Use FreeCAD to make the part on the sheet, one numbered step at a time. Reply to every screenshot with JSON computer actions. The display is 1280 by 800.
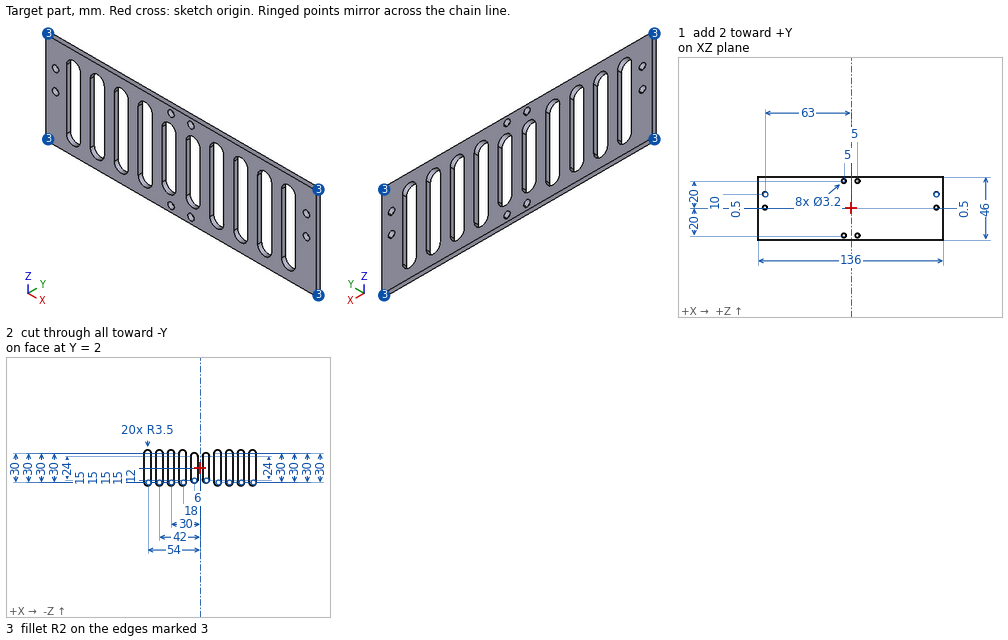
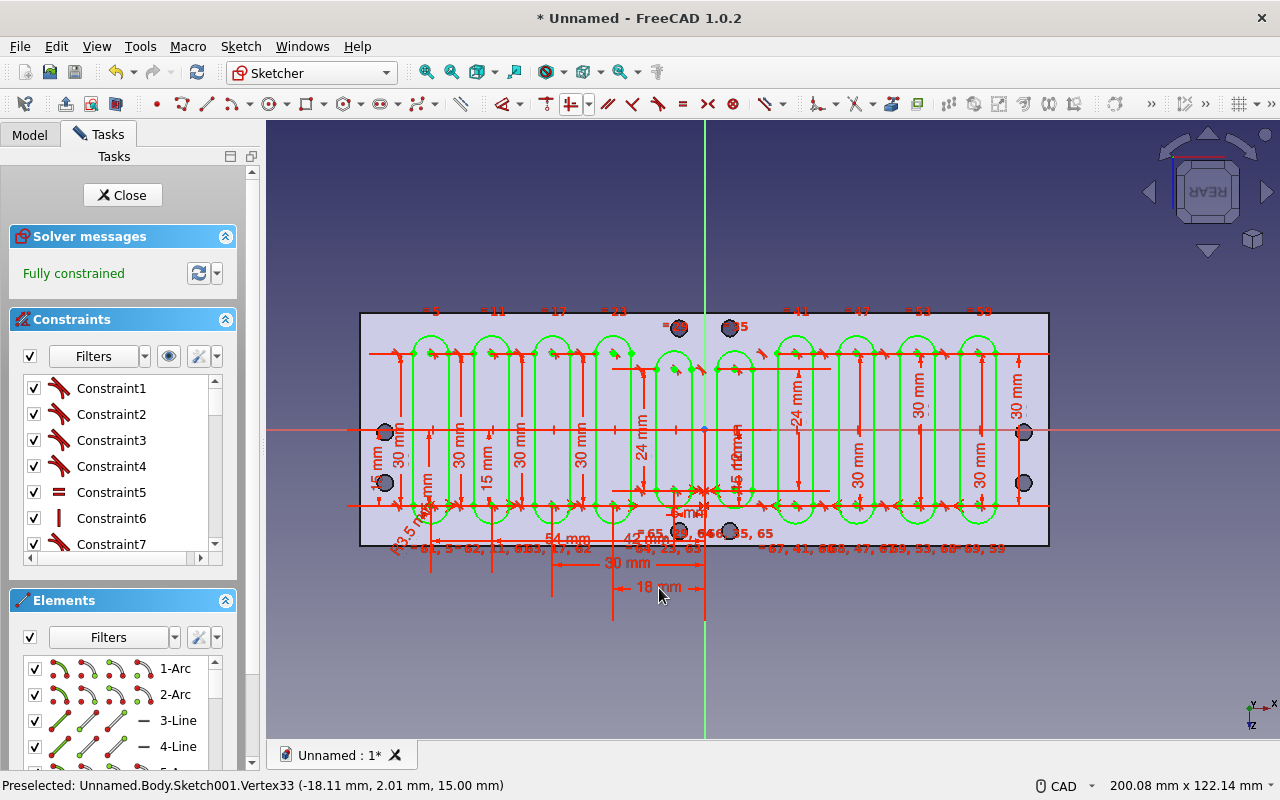
{"action": "left_click", "coordinate": [123, 195]}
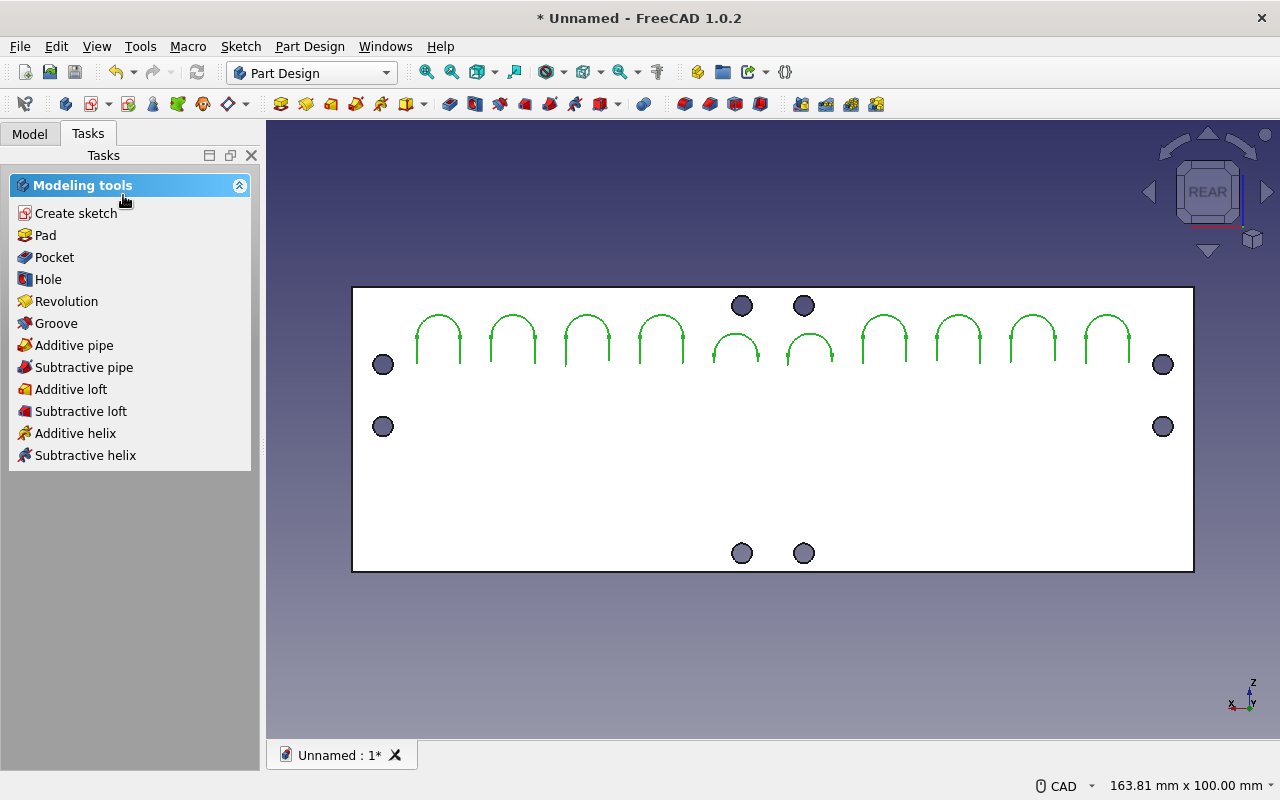
{"action": "left_click", "coordinate": [450, 104]}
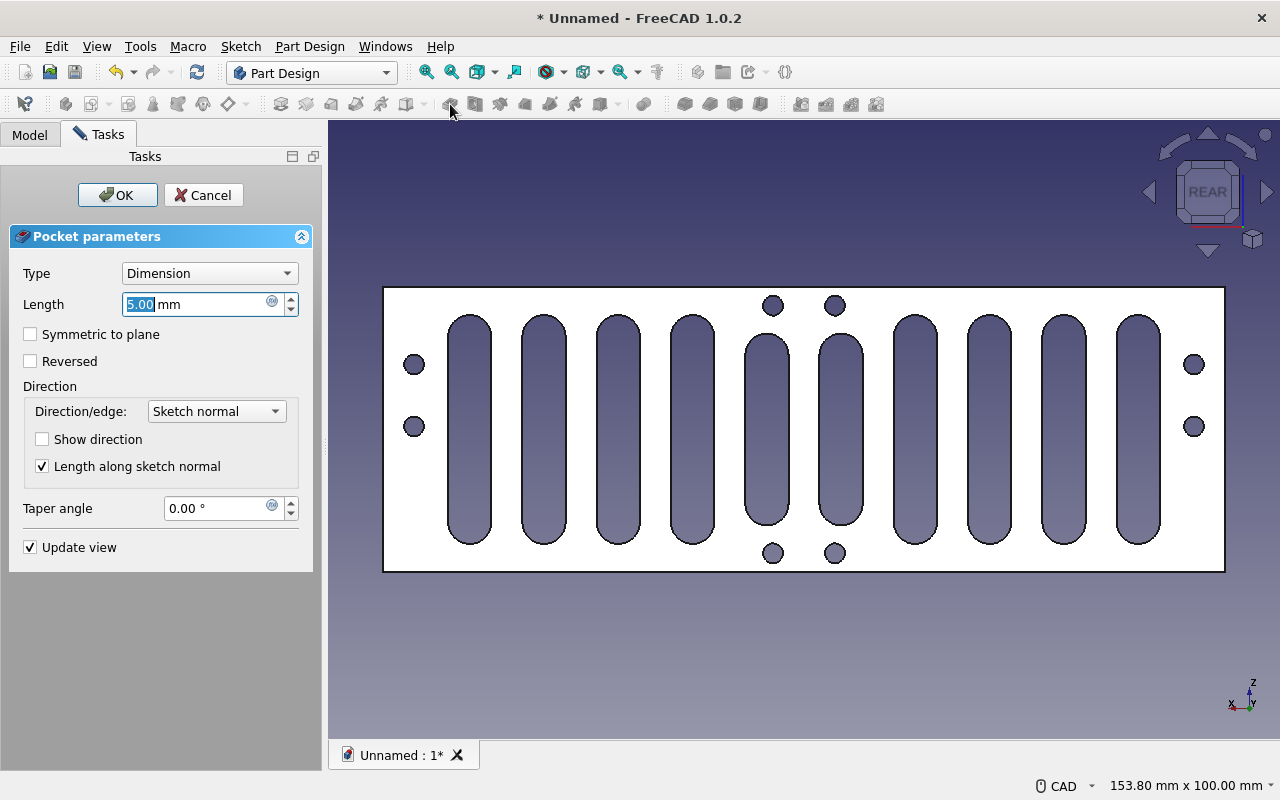
{"action": "left_click", "coordinate": [210, 274]}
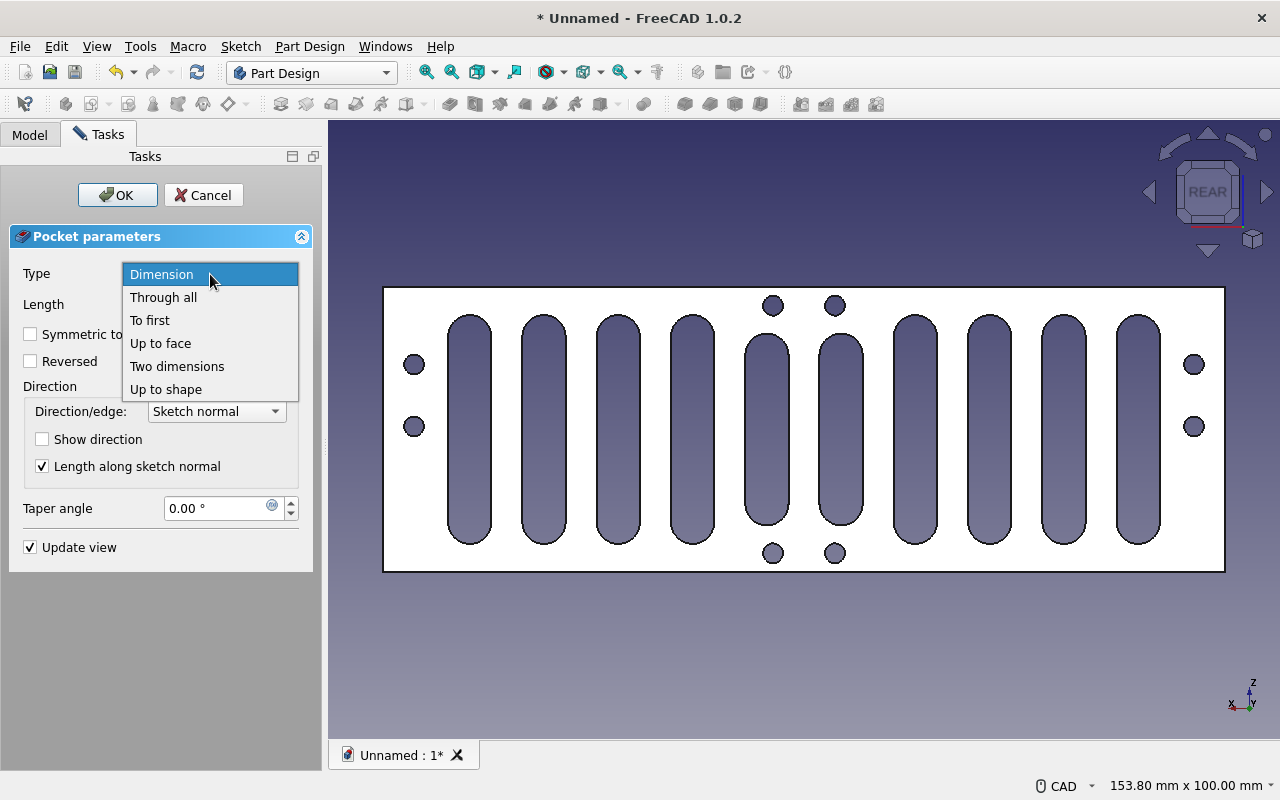
{"action": "left_click", "coordinate": [208, 298]}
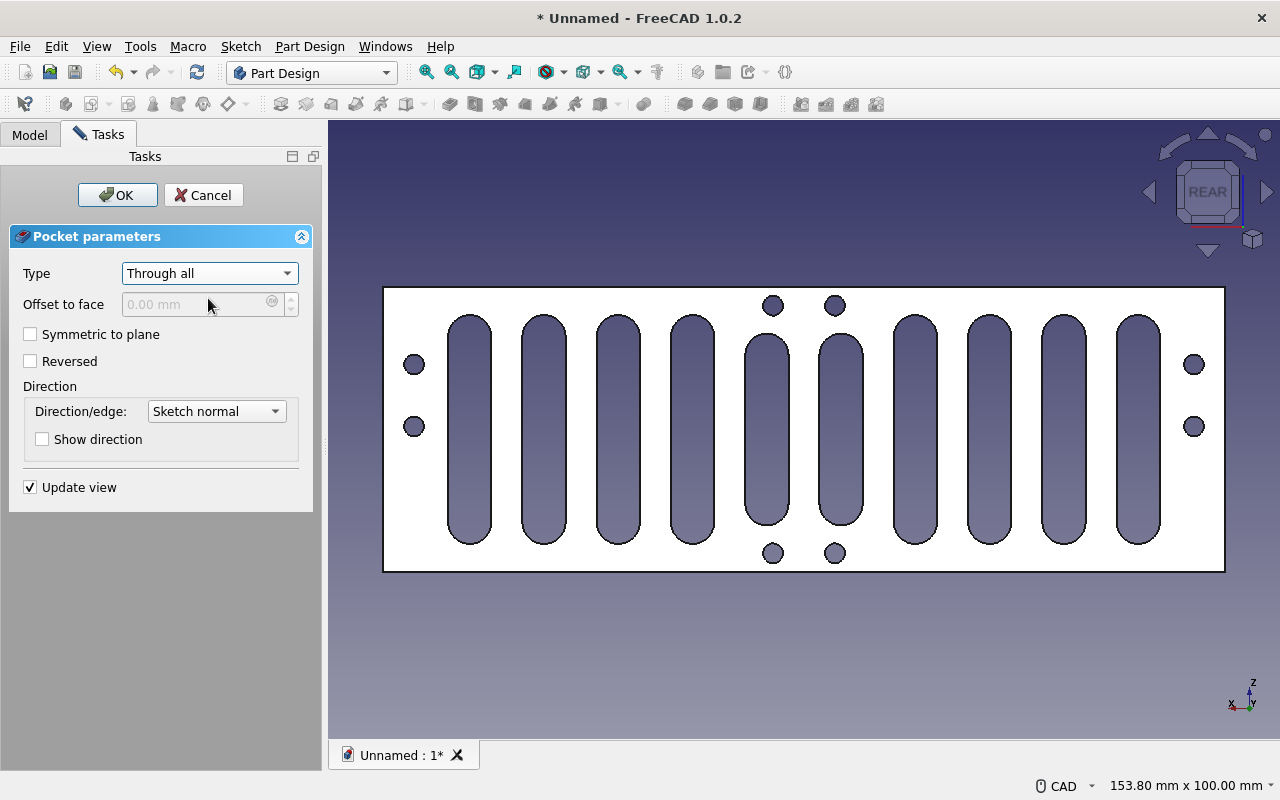
{"action": "left_click", "coordinate": [118, 195]}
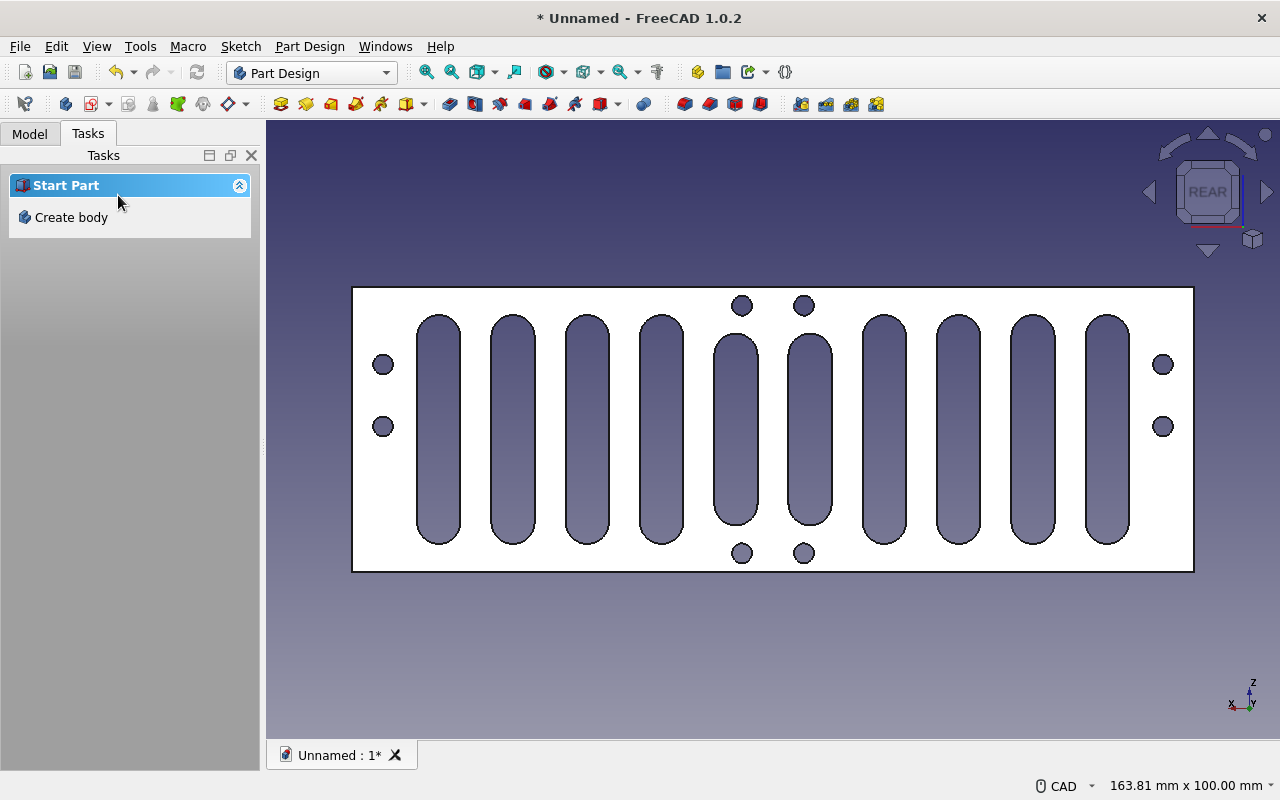
{"action": "key", "text": "0"}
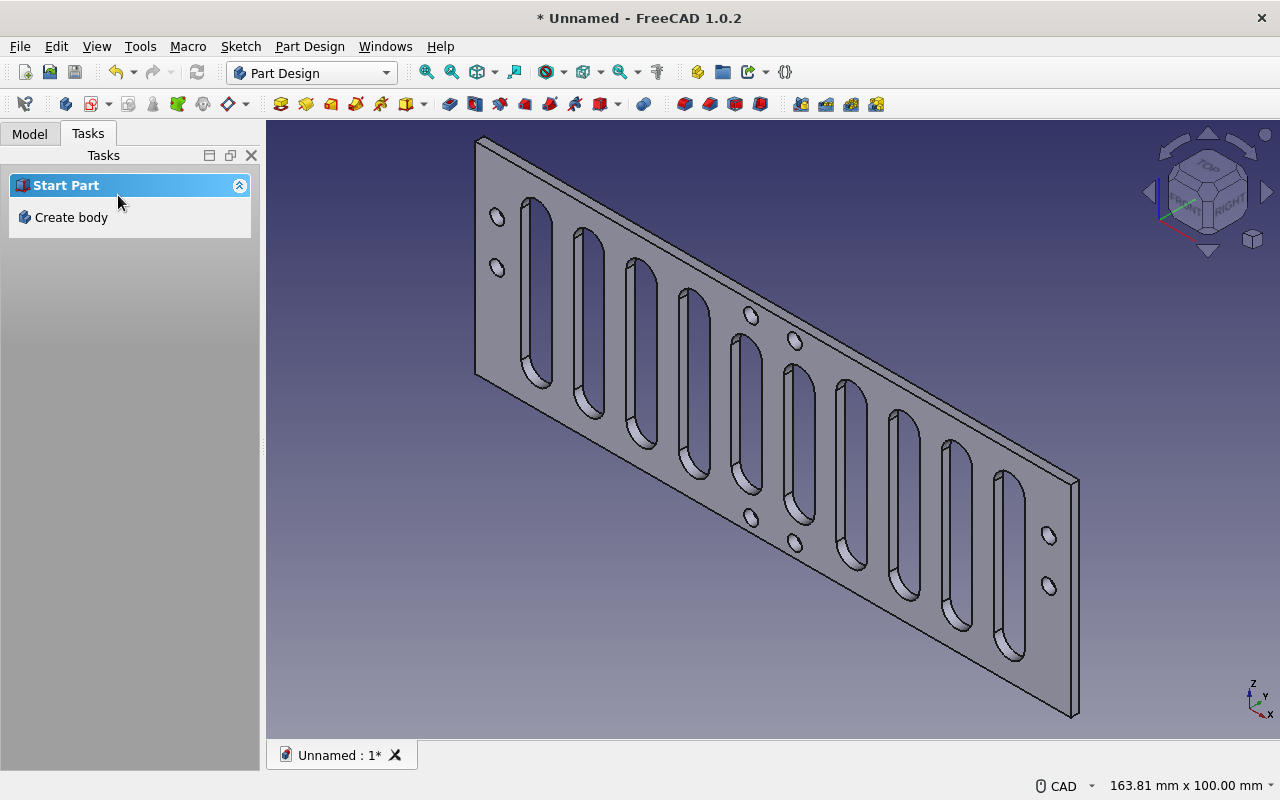
{"action": "left_click", "coordinate": [1077, 481]}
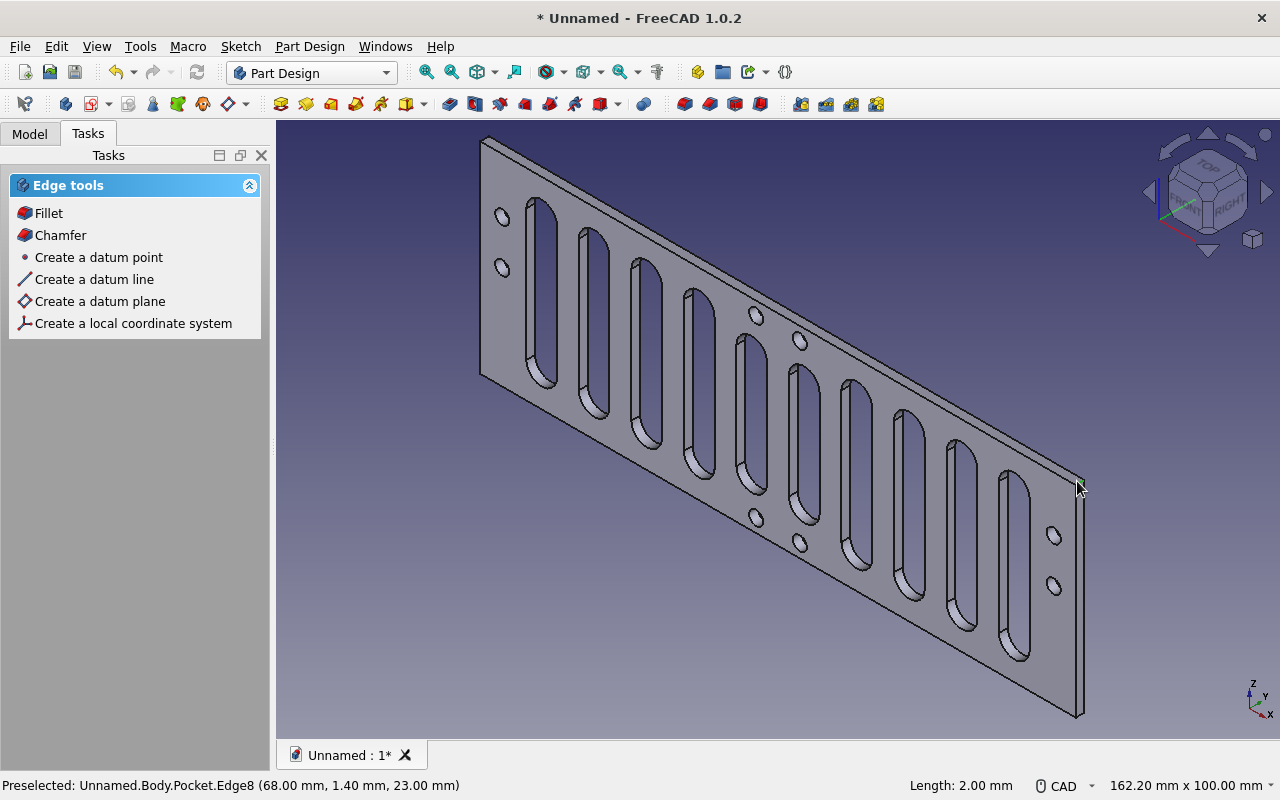
{"action": "scroll", "coordinate": [485, 370], "scroll_direction": "up", "scroll_amount": 6}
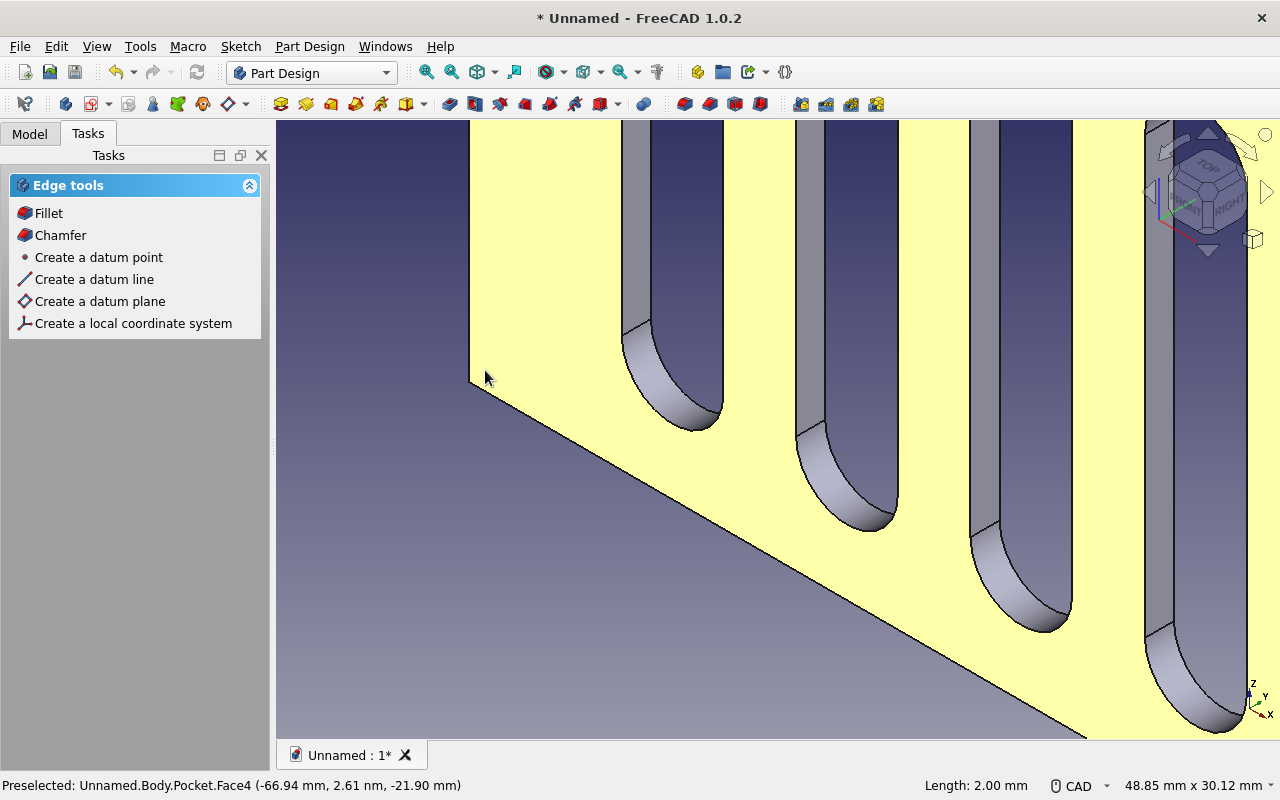
{"action": "left_click", "coordinate": [427, 72]}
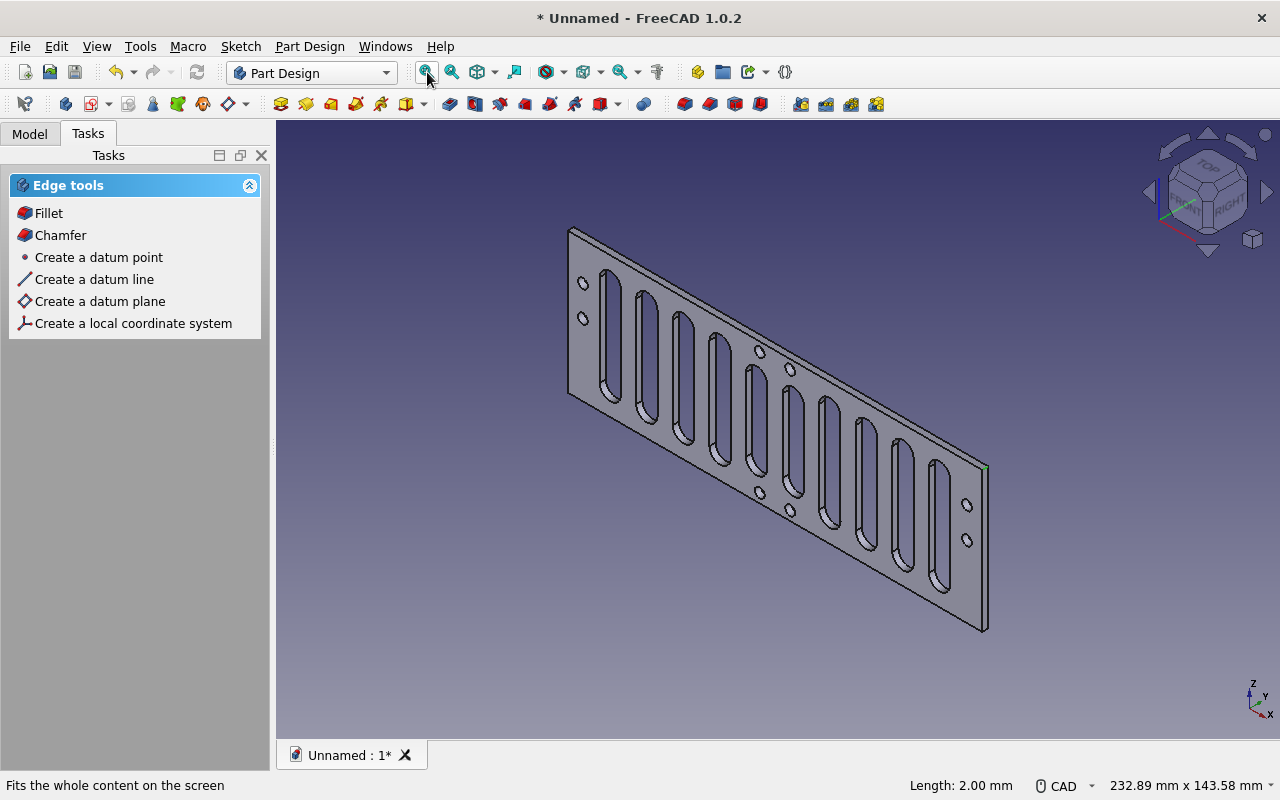
{"action": "key", "text": "2"}